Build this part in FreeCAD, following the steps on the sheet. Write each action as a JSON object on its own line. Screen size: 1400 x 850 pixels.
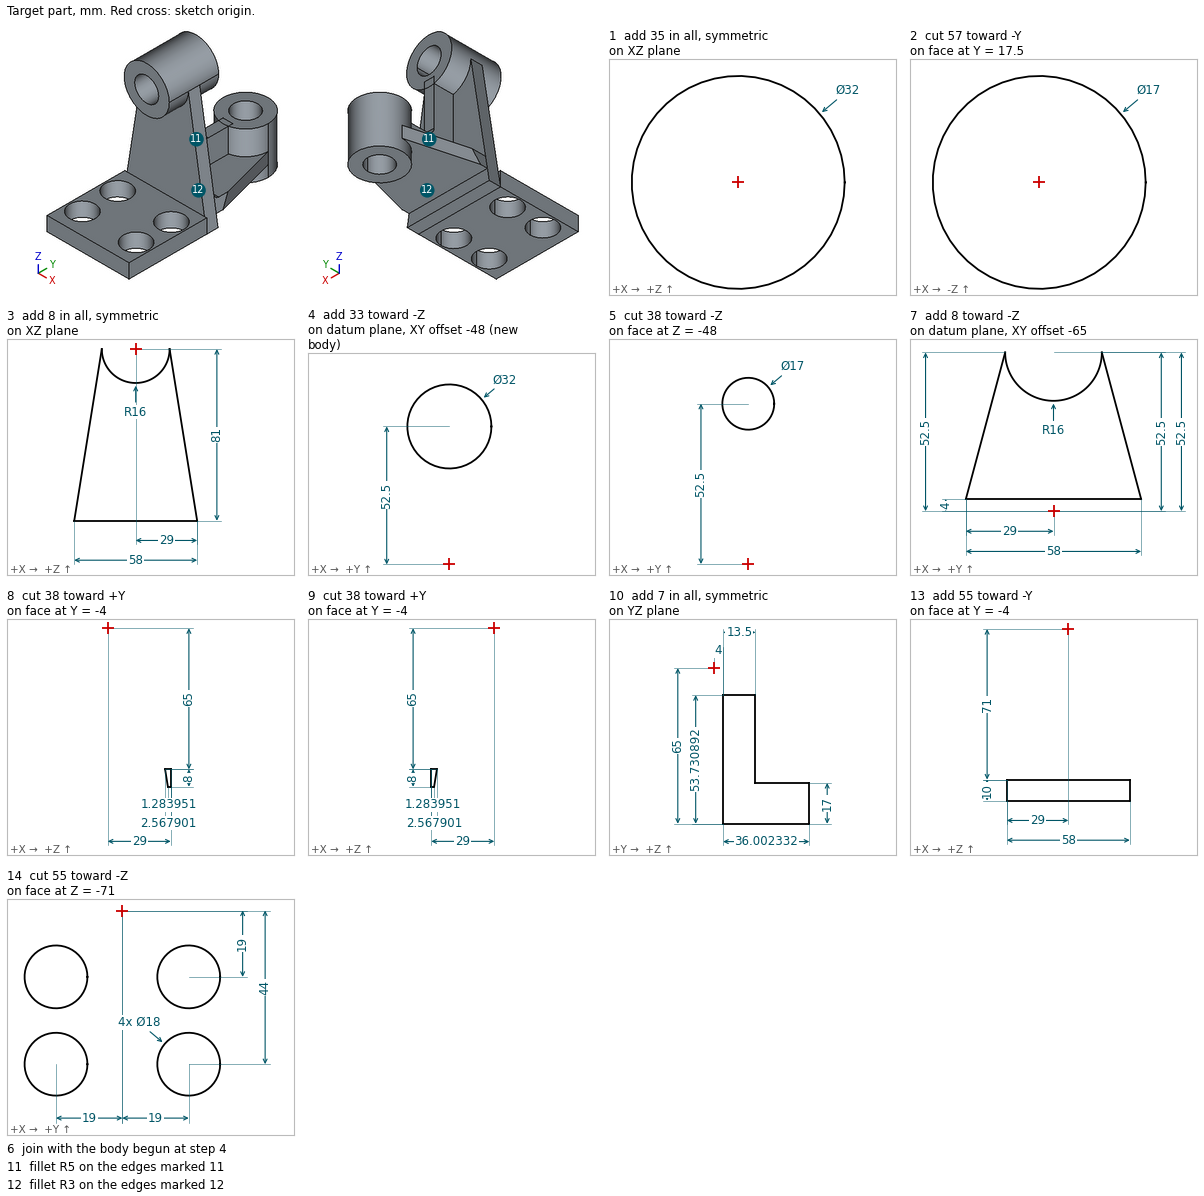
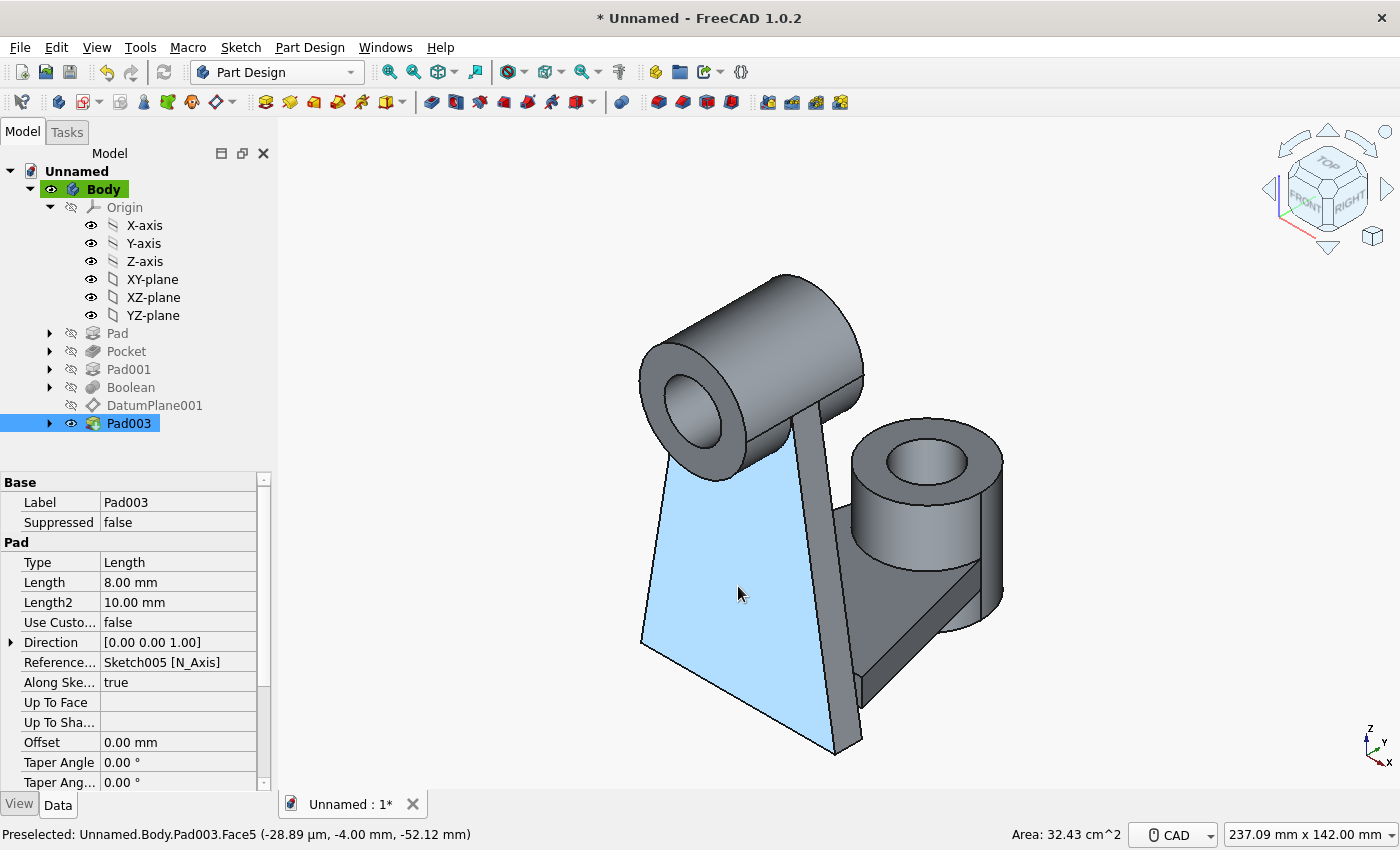
{"action": "left_click", "coordinate": [84, 102]}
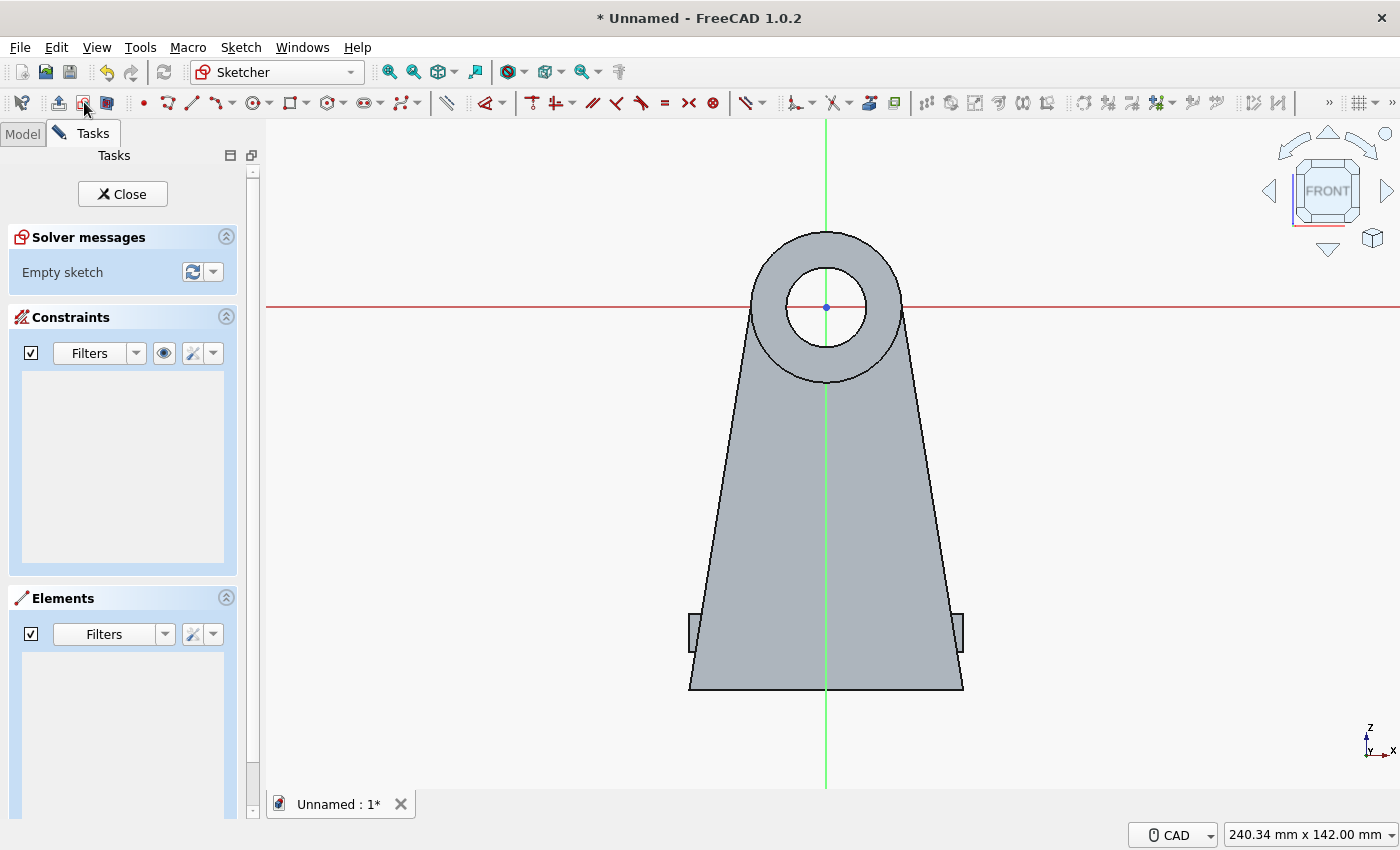
{"action": "scroll", "coordinate": [976, 651], "scroll_direction": "up", "scroll_amount": 12}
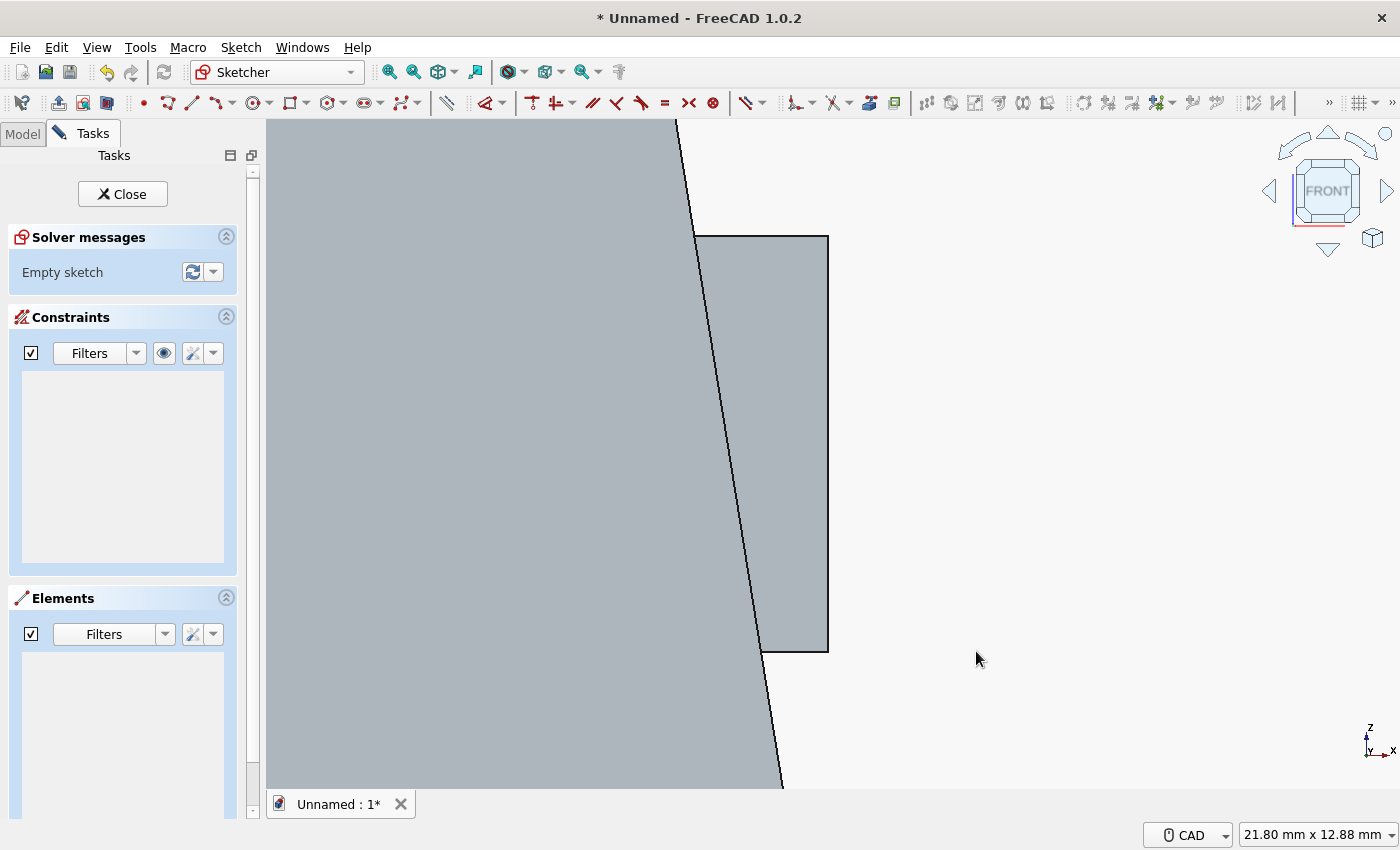
{"action": "key", "text": "g m"}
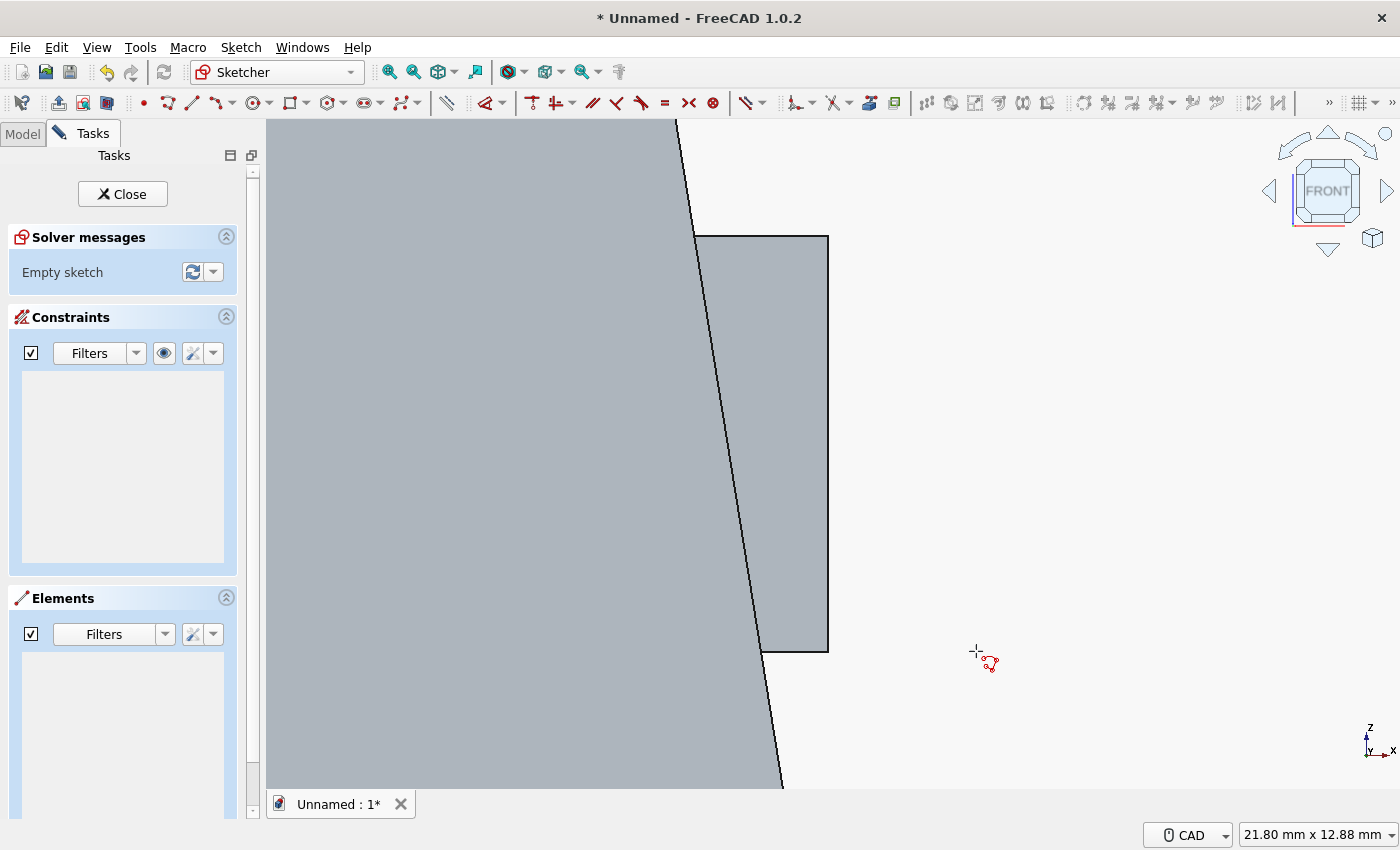
{"action": "left_click", "coordinate": [694, 236]}
{"action": "left_click", "coordinate": [761, 652]}
{"action": "left_click", "coordinate": [828, 652]}
{"action": "left_click", "coordinate": [828, 236]}
{"action": "left_click", "coordinate": [694, 237]}
{"action": "key", "text": "Escape"}
{"action": "key", "text": "Escape"}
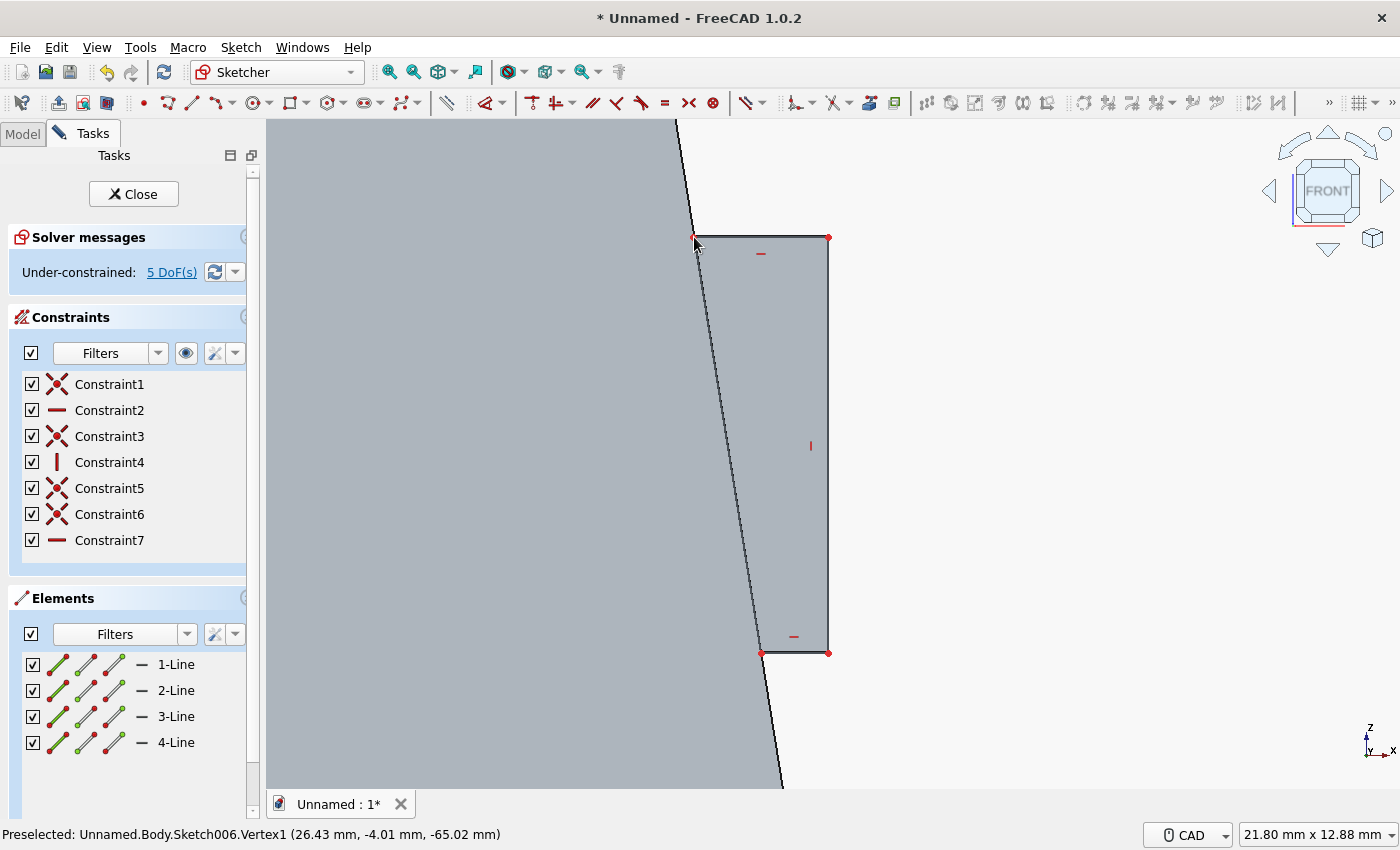
{"action": "key", "text": "d"}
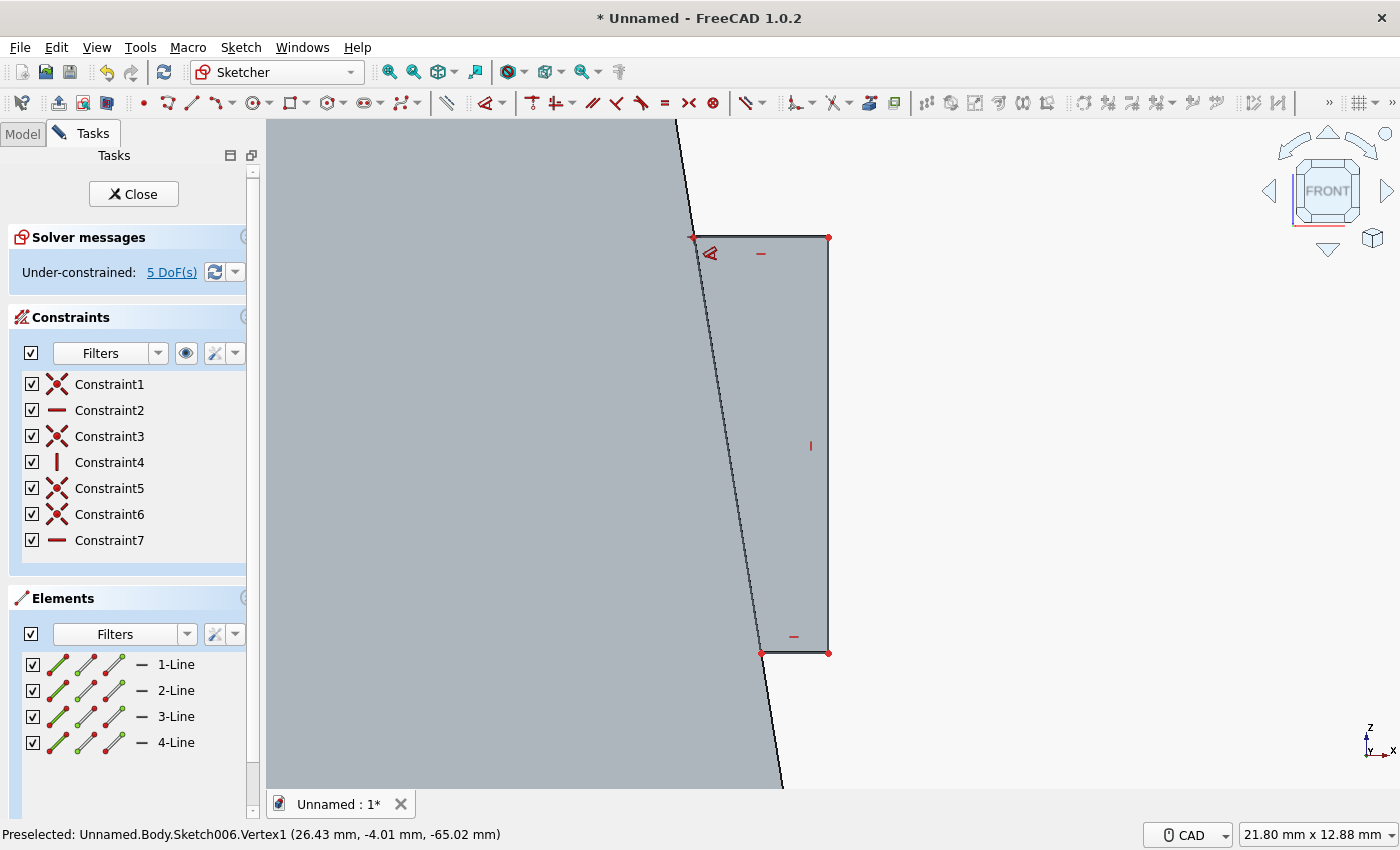
{"action": "left_click", "coordinate": [828, 528]}
{"action": "left_click", "coordinate": [862, 445]}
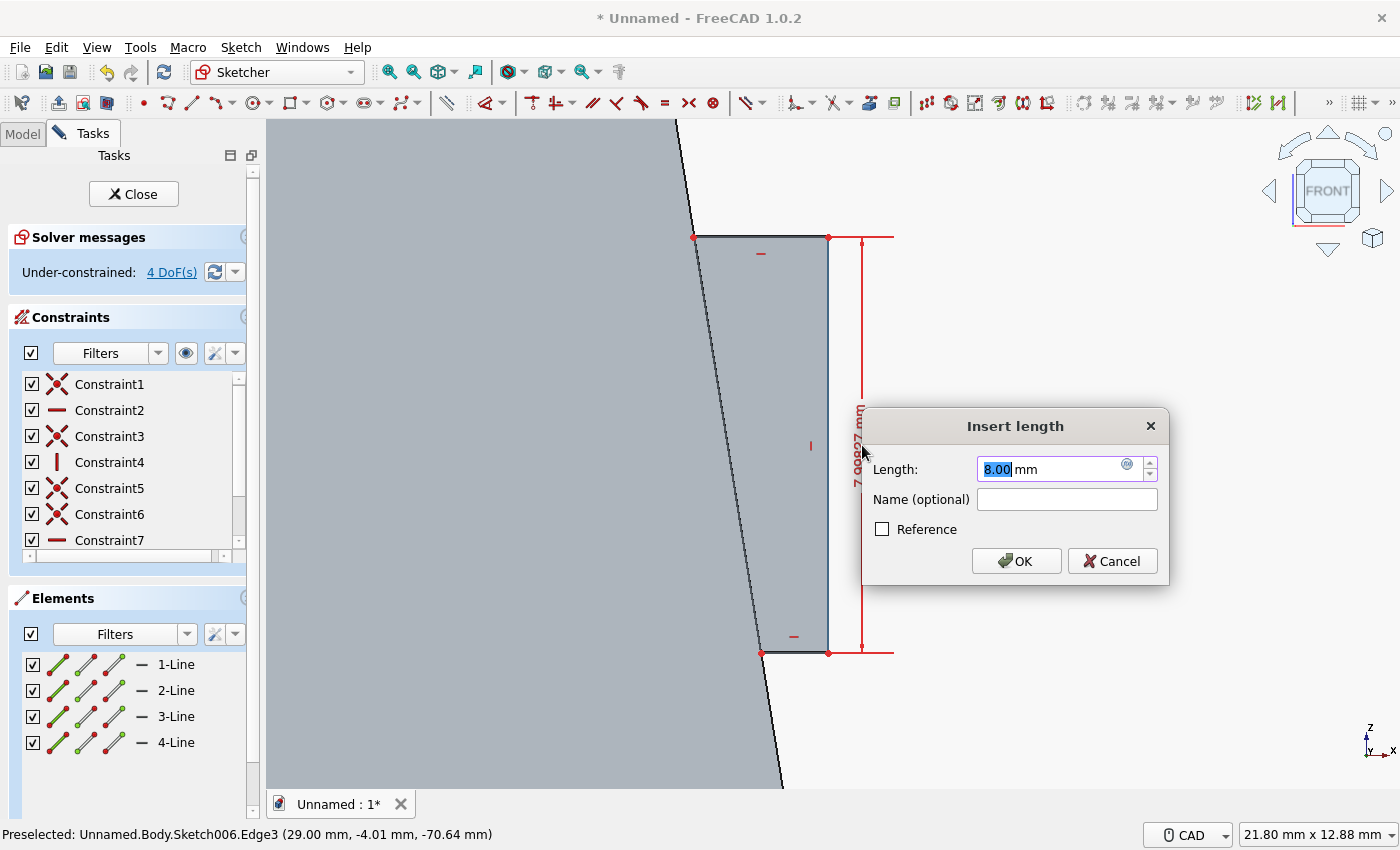
{"action": "type", "text": "8"}
{"action": "key", "text": "Return"}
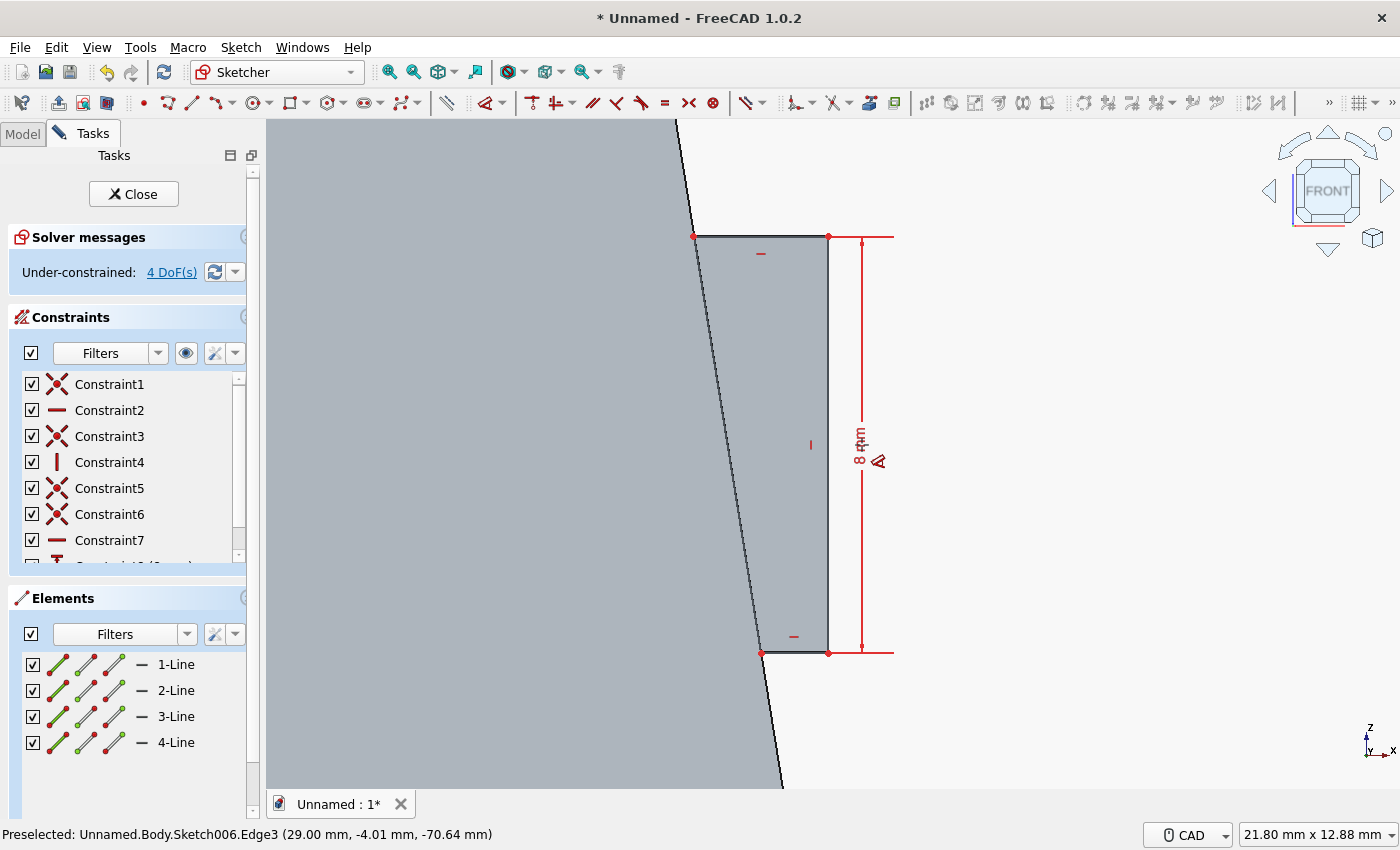
{"action": "left_click", "coordinate": [694, 237]}
{"action": "left_click", "coordinate": [728, 192]}